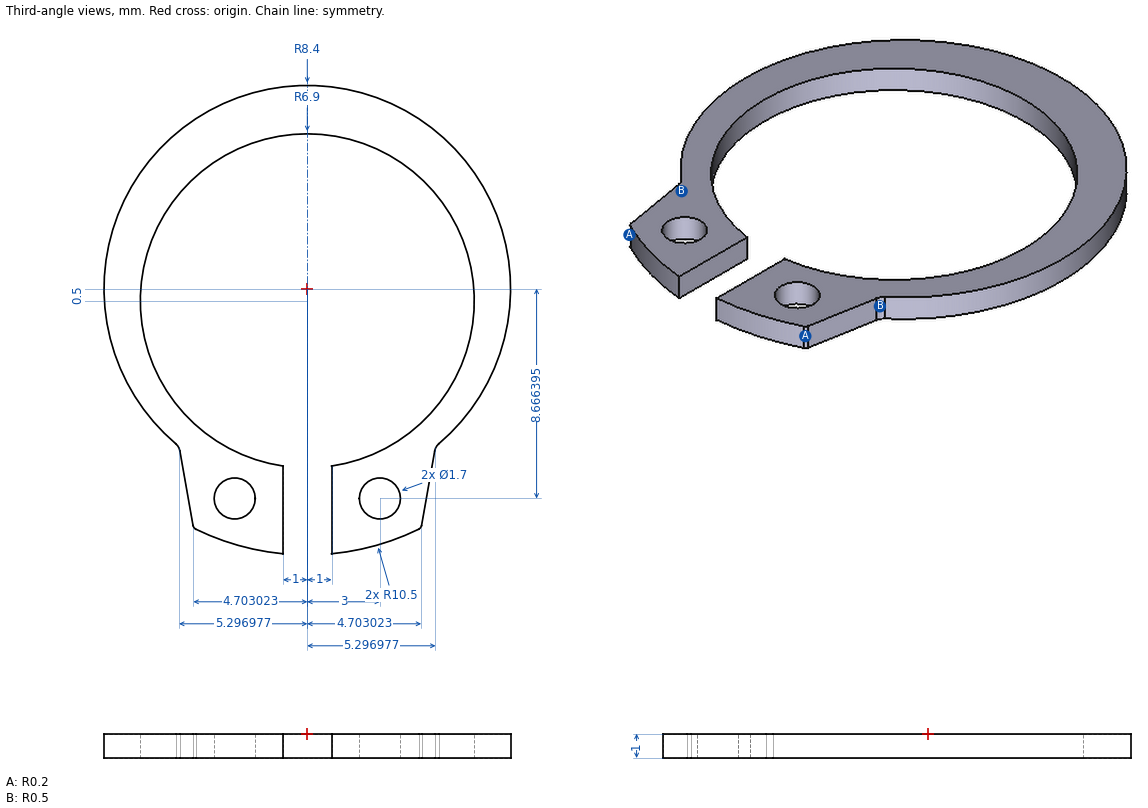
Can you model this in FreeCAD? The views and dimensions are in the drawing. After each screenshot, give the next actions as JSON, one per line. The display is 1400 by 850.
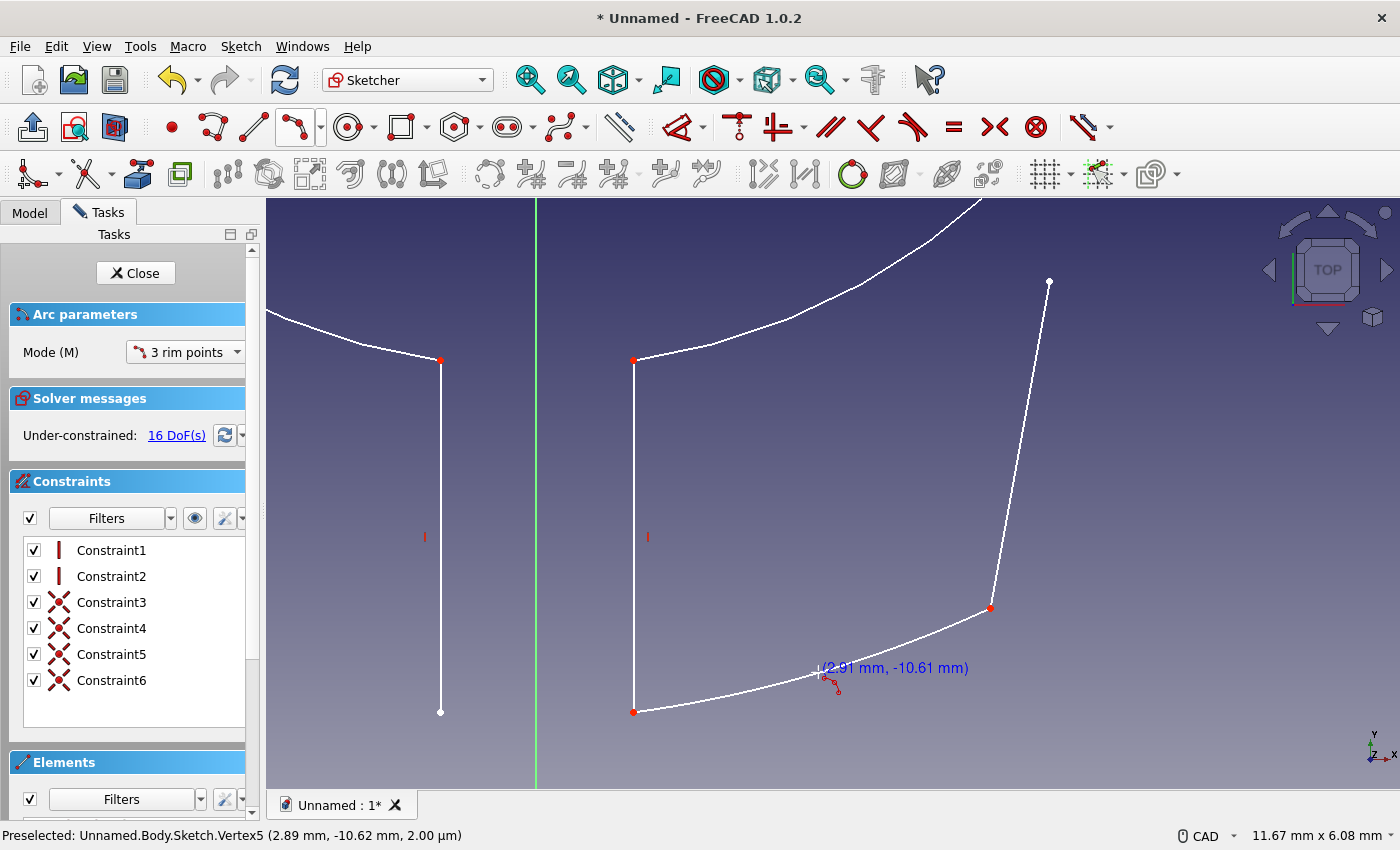
{"action": "scroll", "coordinate": [822, 677], "scroll_direction": "down", "scroll_amount": 8}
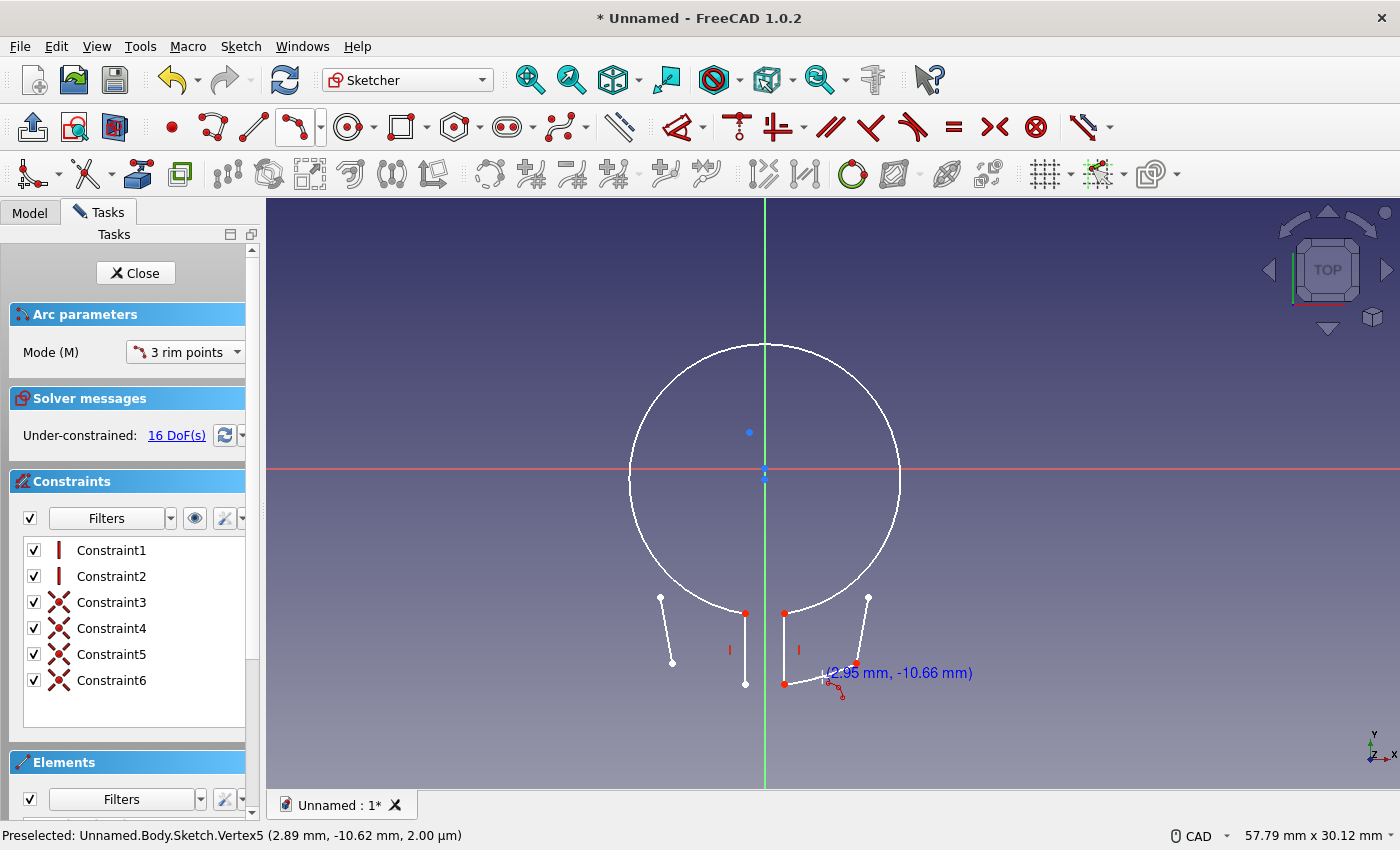
{"action": "left_click", "coordinate": [868, 598]}
{"action": "left_click", "coordinate": [660, 598]}
{"action": "left_click", "coordinate": [842, 323]}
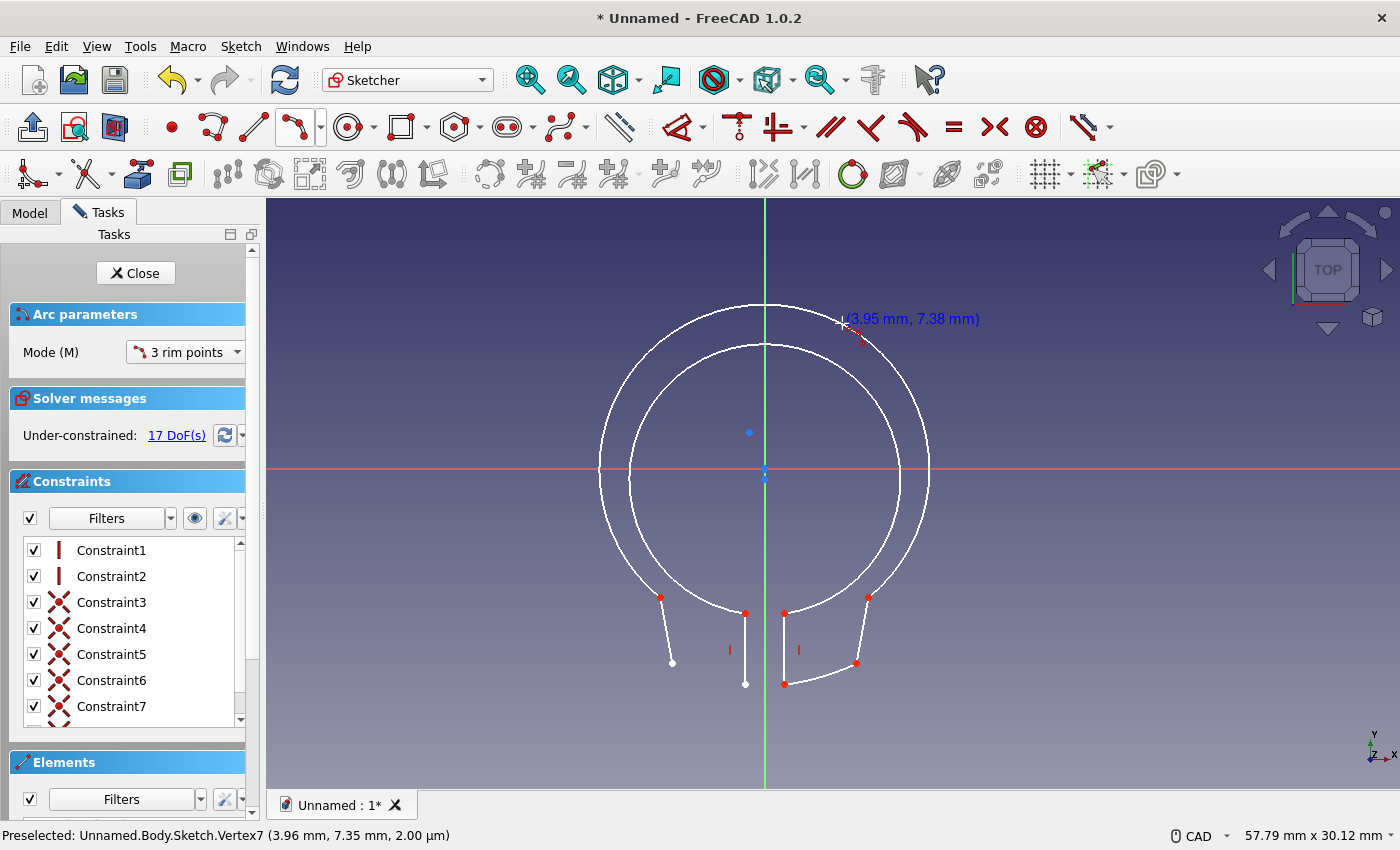
{"action": "left_click", "coordinate": [672, 664]}
{"action": "left_click", "coordinate": [745, 685]}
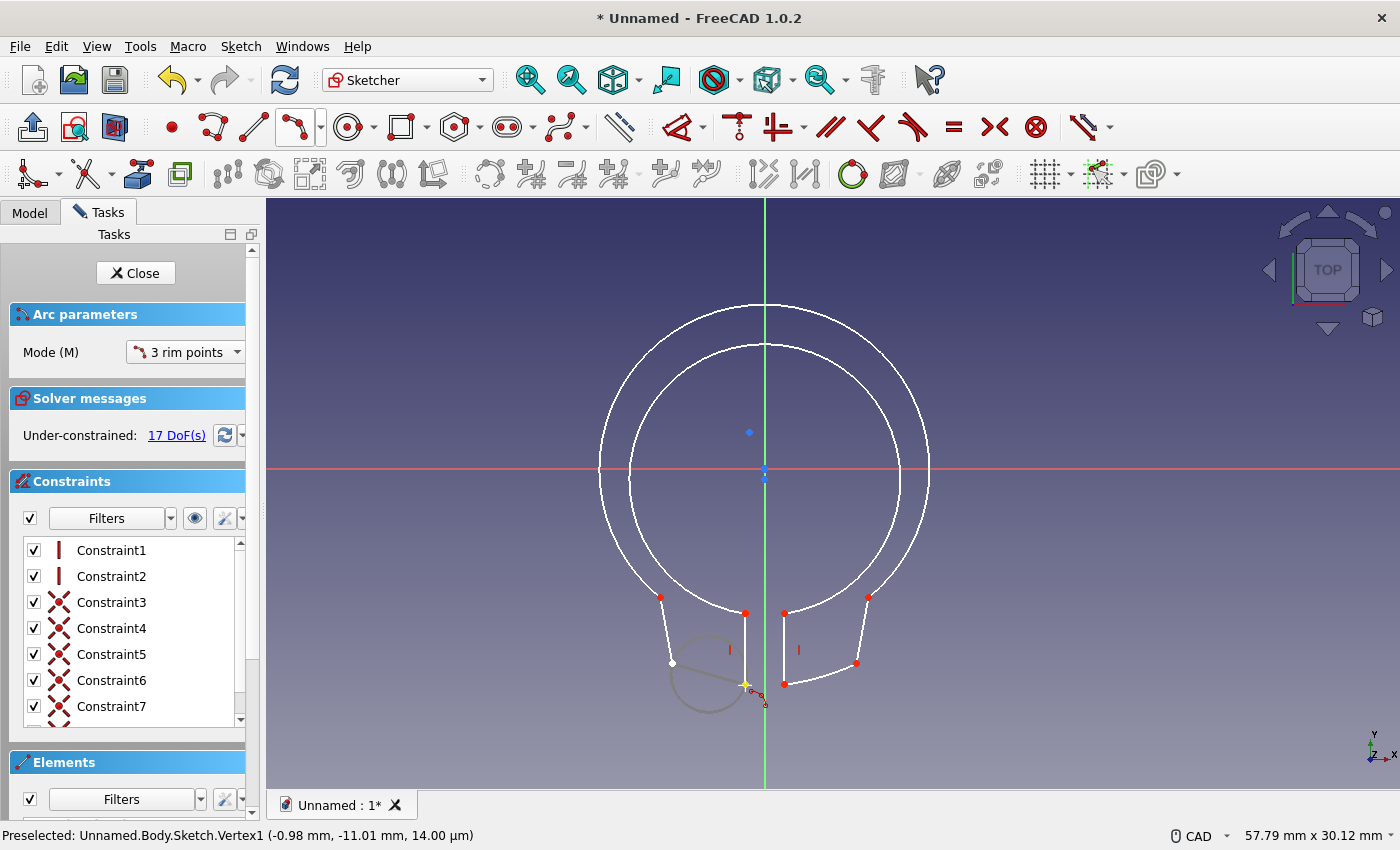
{"action": "scroll", "coordinate": [708, 677], "scroll_direction": "up", "scroll_amount": 8}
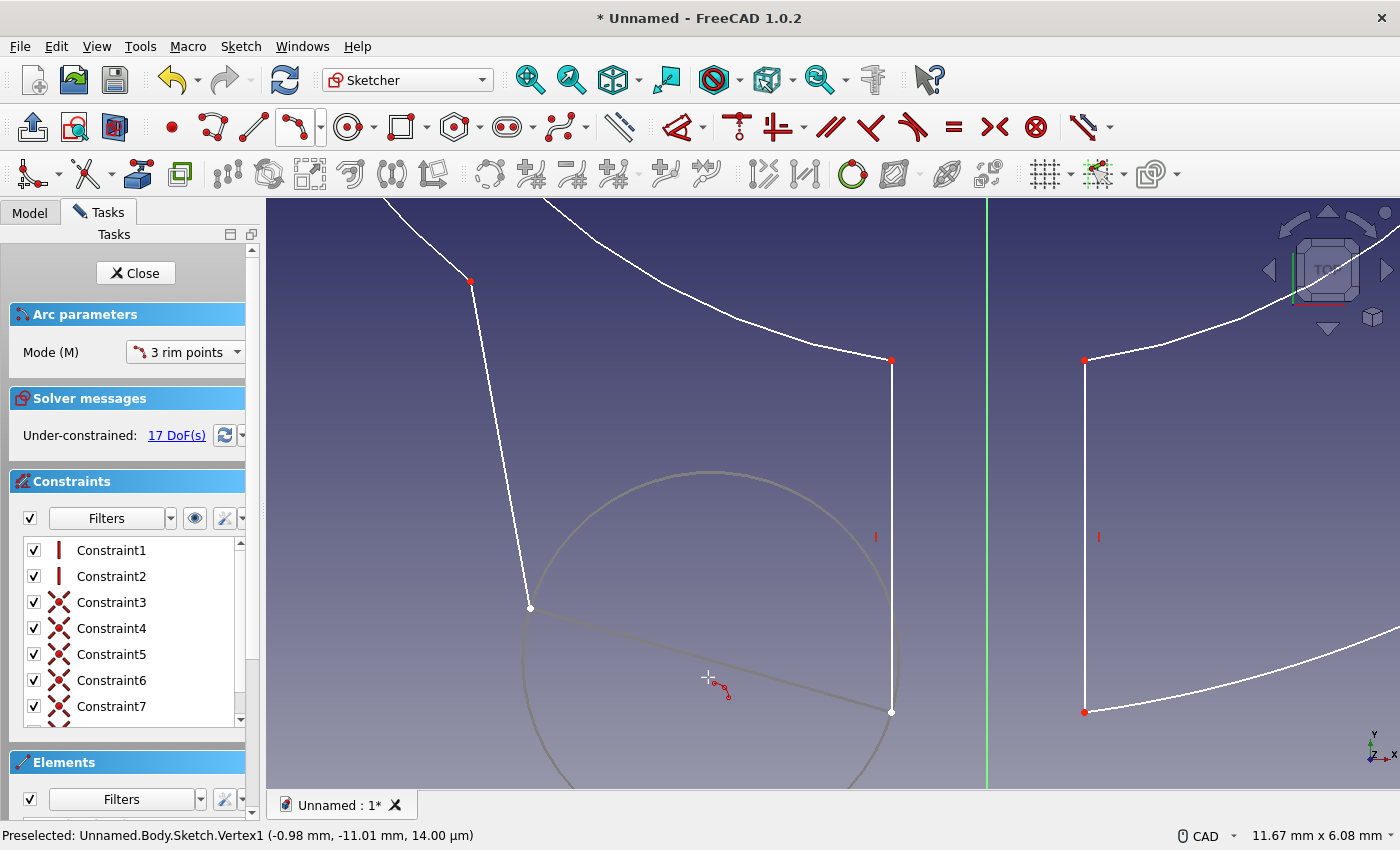
{"action": "left_click", "coordinate": [705, 672]}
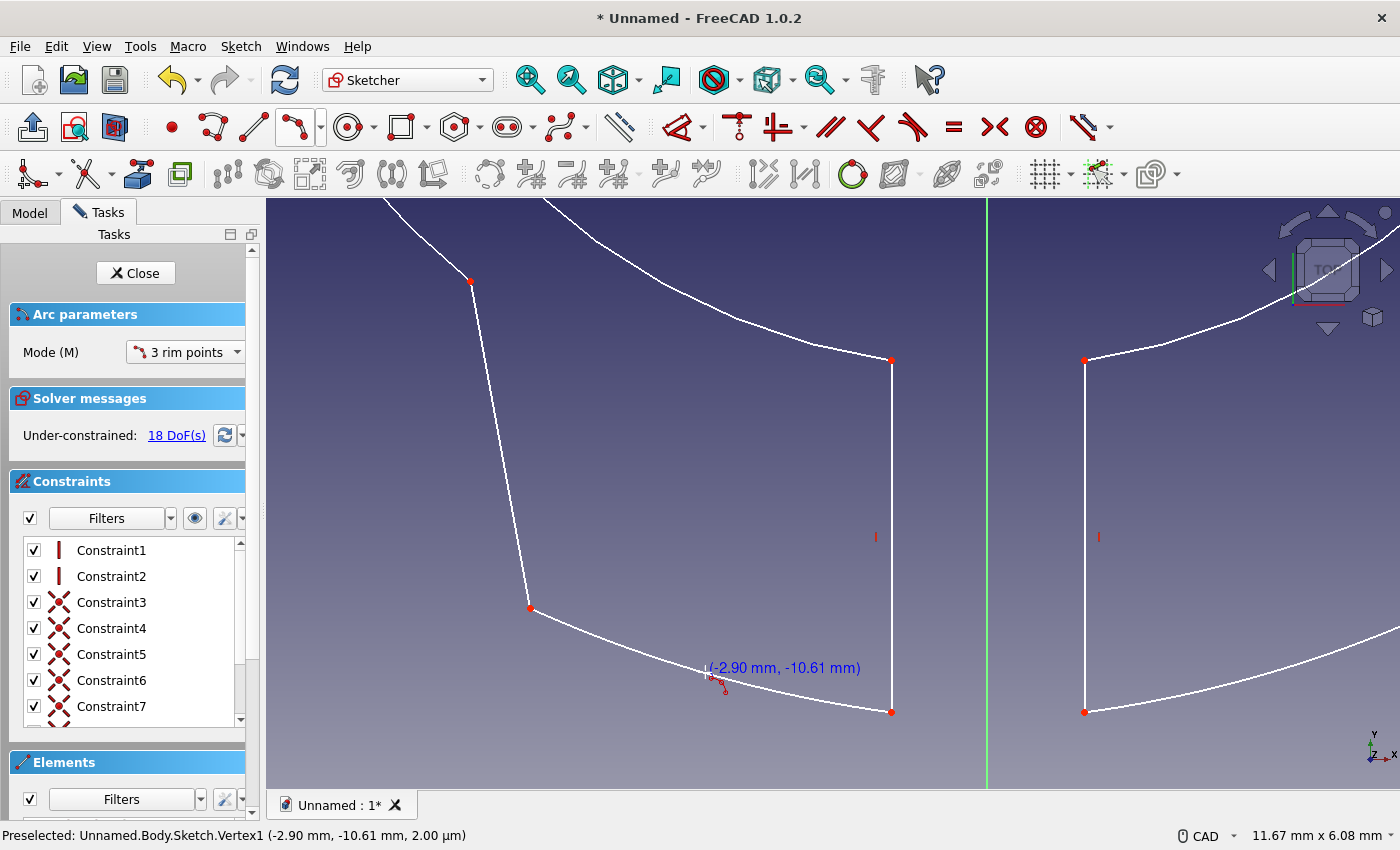
{"action": "left_click", "coordinate": [348, 128]}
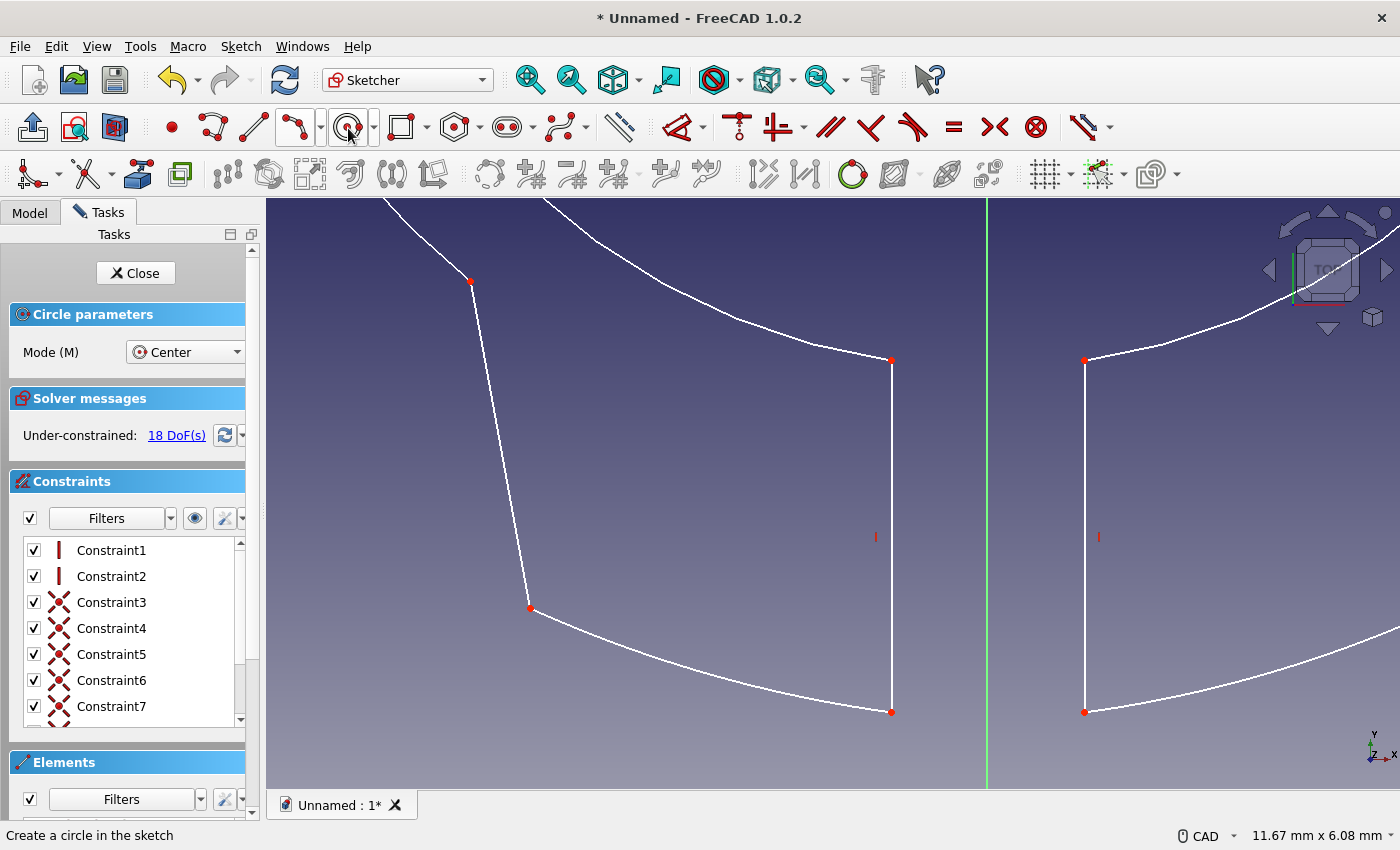
{"action": "scroll", "coordinate": [708, 677], "scroll_direction": "down", "scroll_amount": 8}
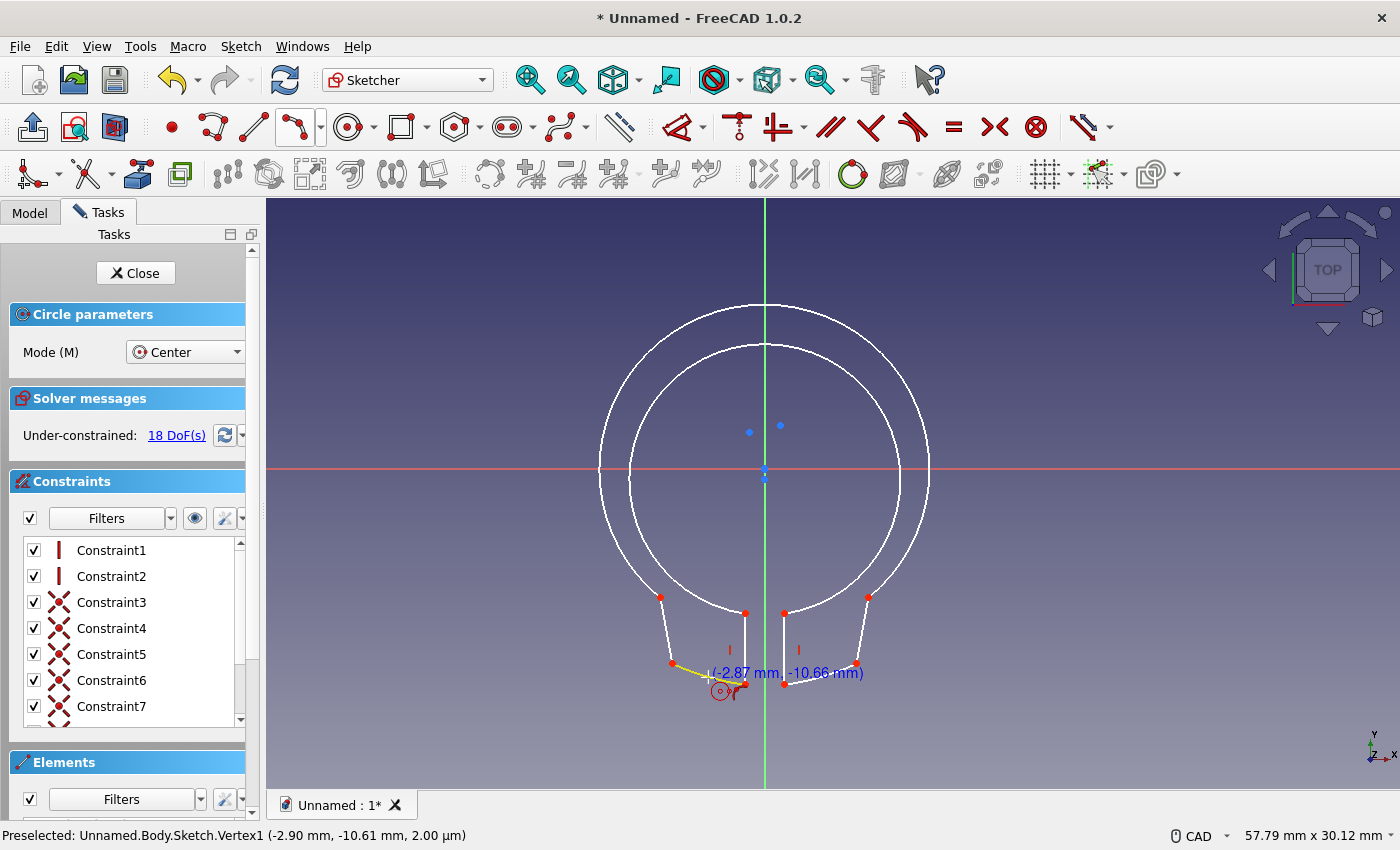
{"action": "scroll", "coordinate": [823, 639], "scroll_direction": "up", "scroll_amount": 2}